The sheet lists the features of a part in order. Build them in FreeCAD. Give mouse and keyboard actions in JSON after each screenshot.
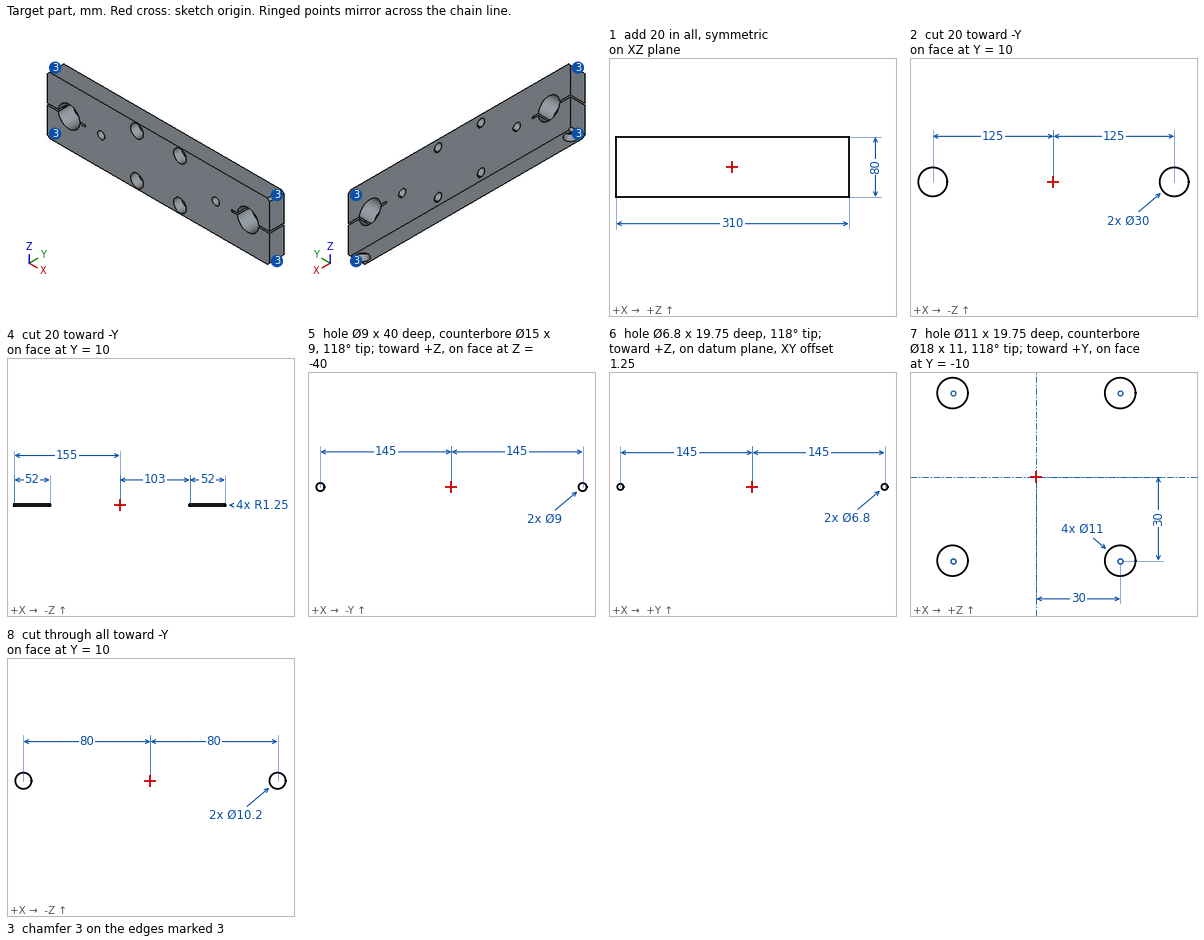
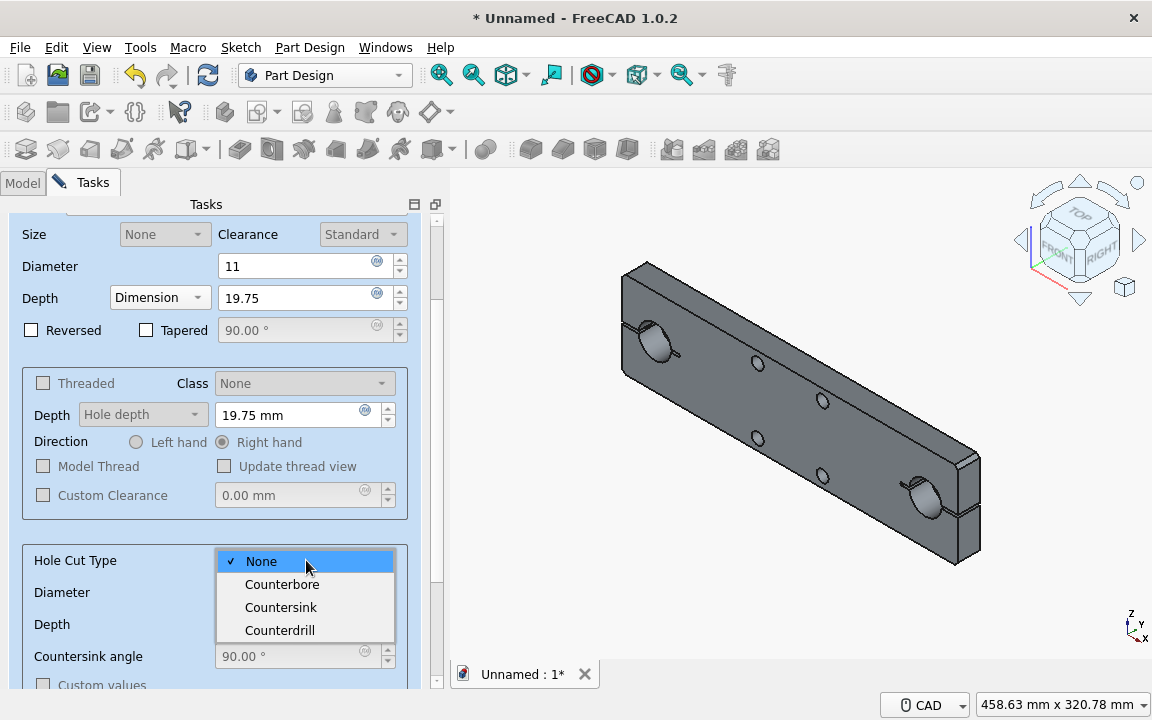
{"action": "left_click", "coordinate": [304, 584]}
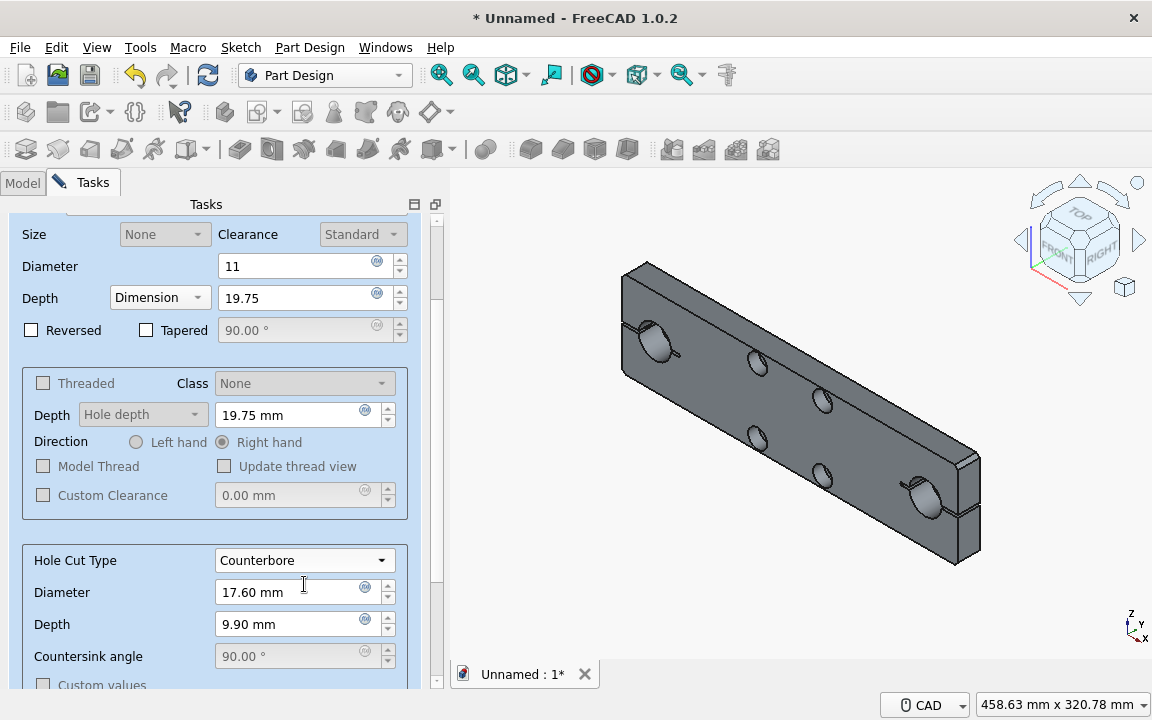
{"action": "triple_click", "coordinate": [298, 592]}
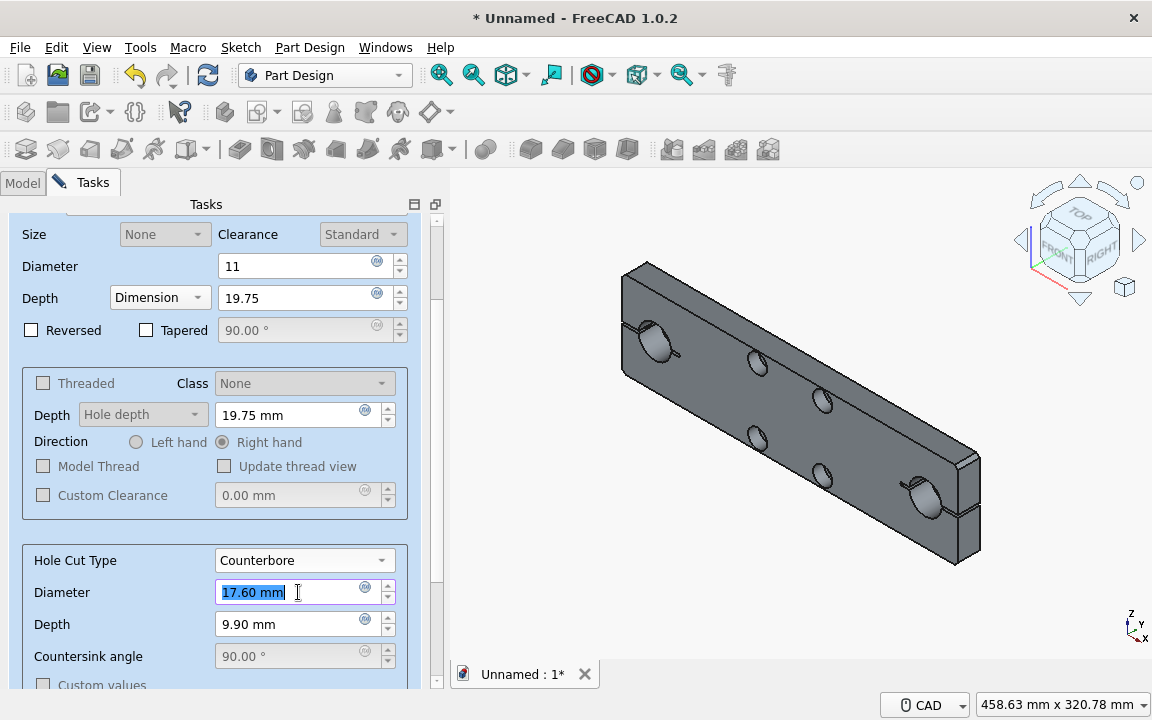
{"action": "type", "text": "18"}
{"action": "key", "text": "Tab"}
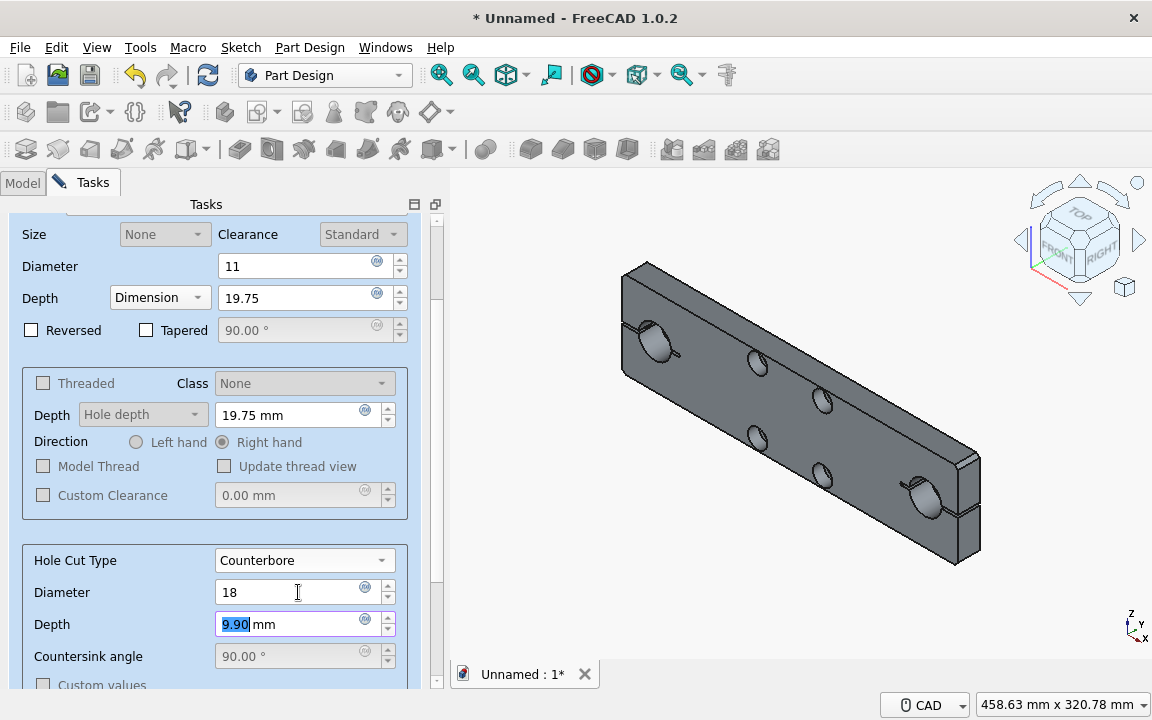
{"action": "type", "text": "11"}
{"action": "key", "text": "Tab"}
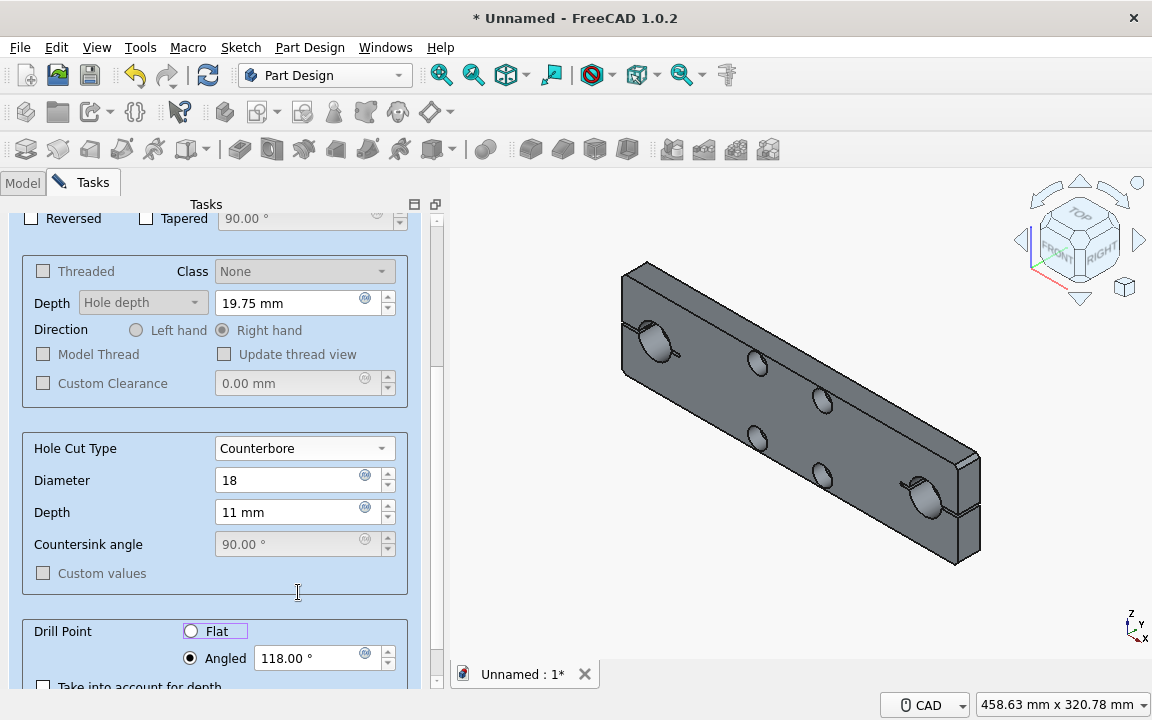
{"action": "scroll", "coordinate": [437, 451], "scroll_direction": "up", "scroll_amount": 5}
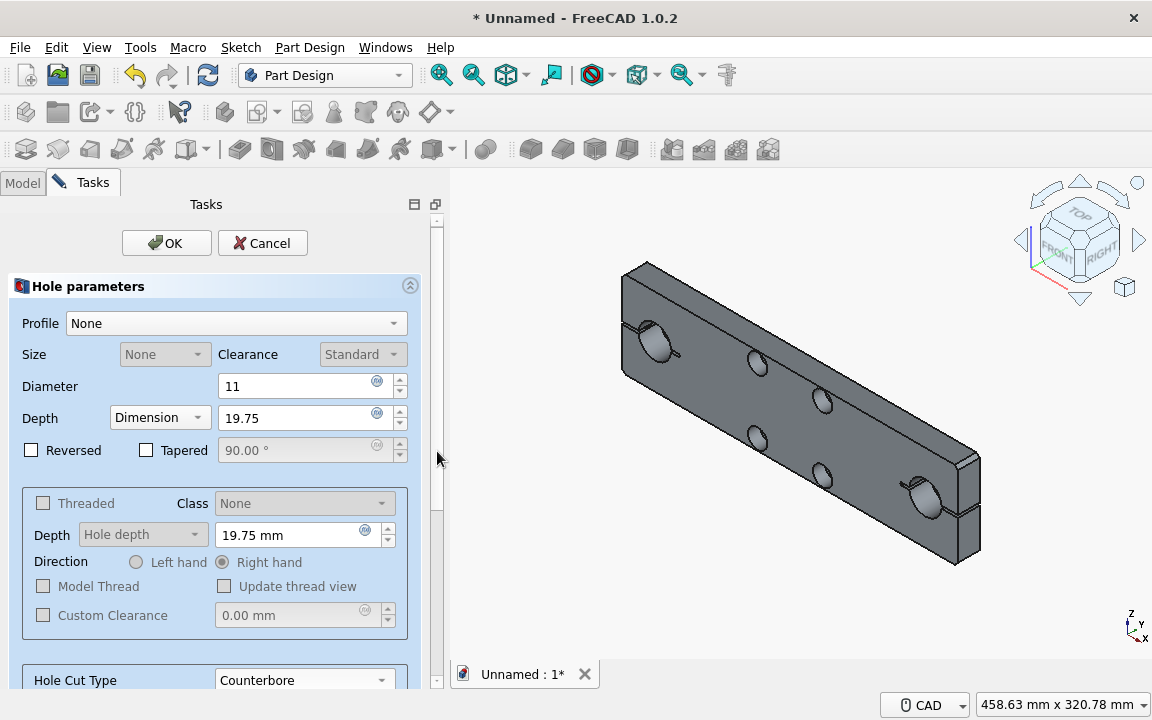
{"action": "left_click", "coordinate": [167, 243]}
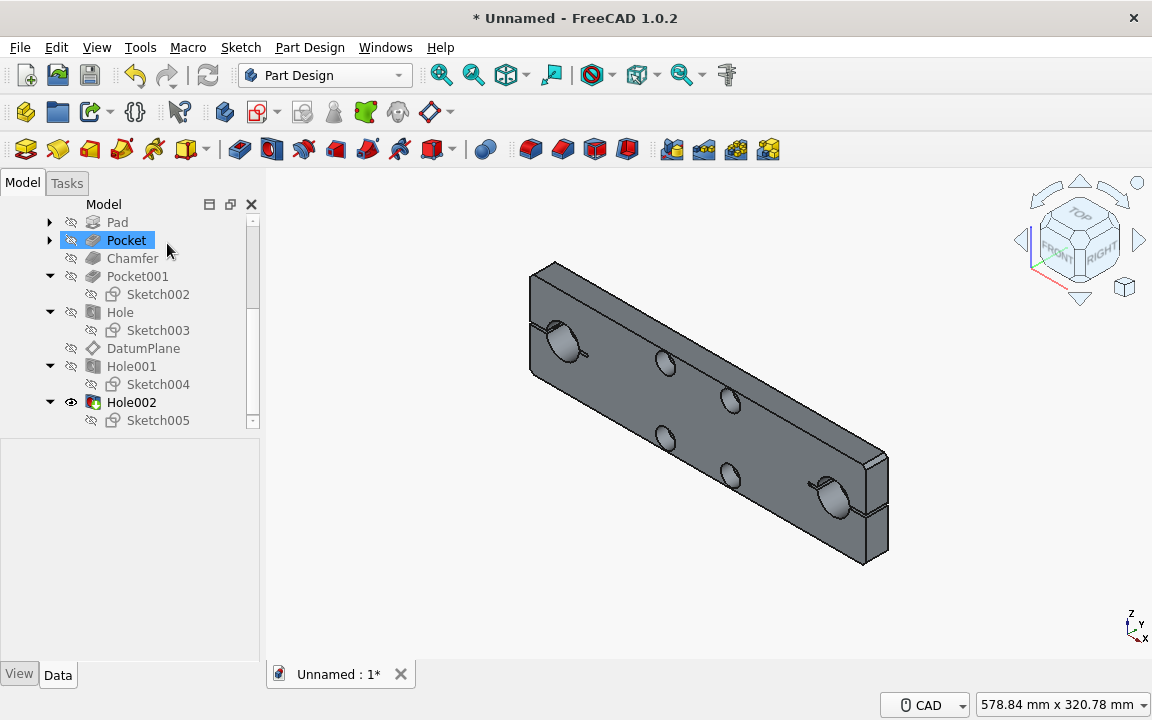
{"action": "key", "text": "4"}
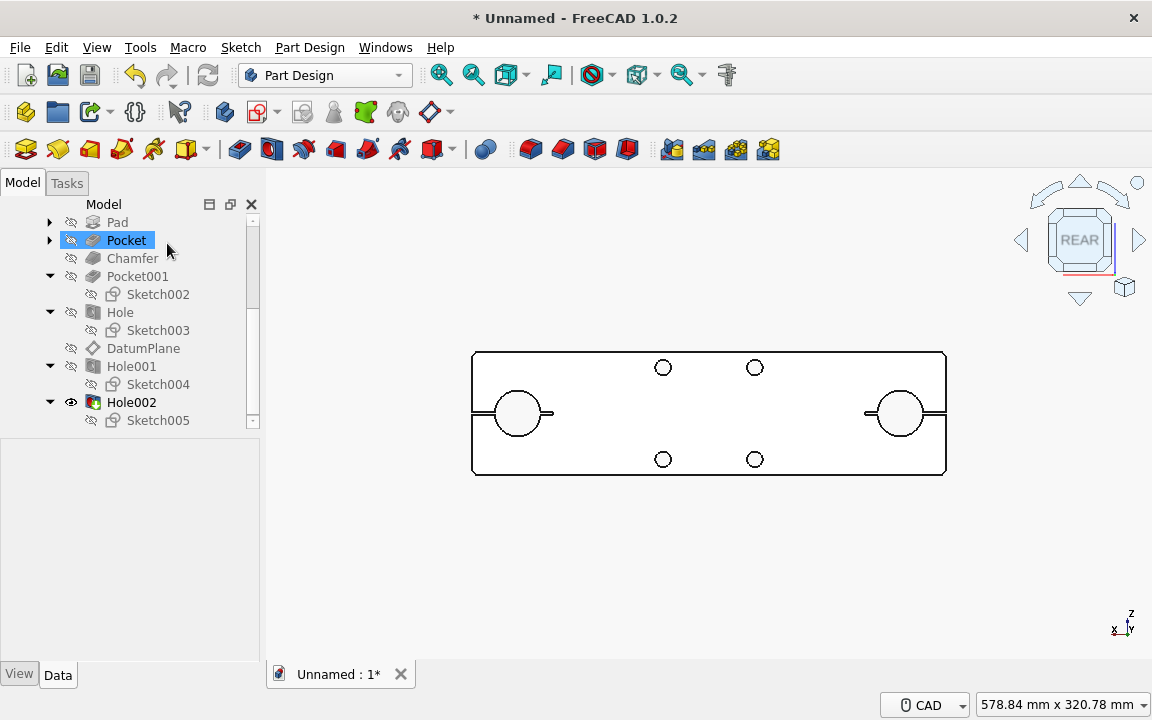
{"action": "left_click", "coordinate": [709, 412]}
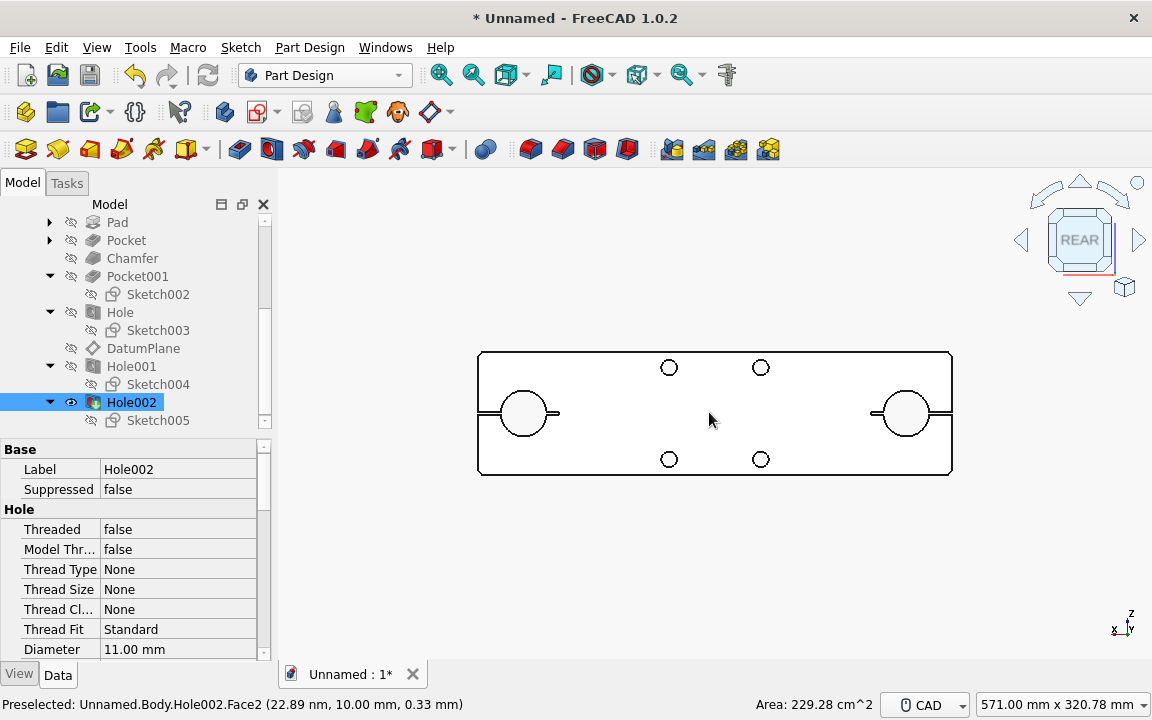
{"action": "left_click", "coordinate": [258, 112]}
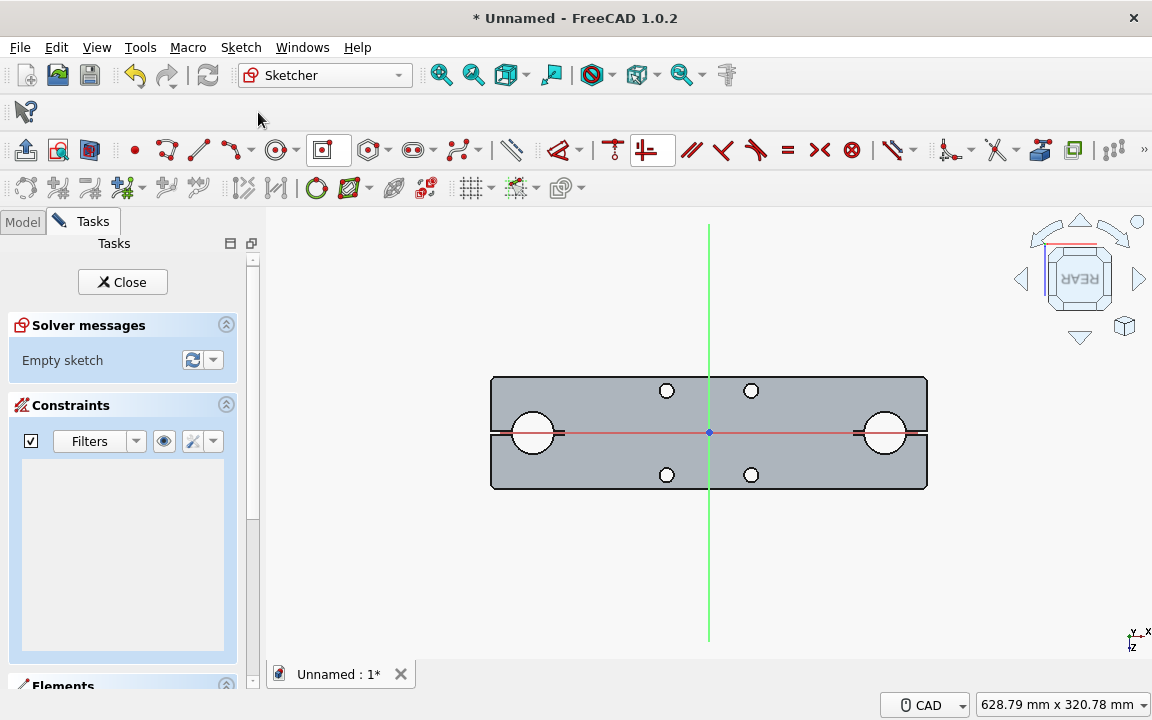
{"action": "scroll", "coordinate": [765, 433], "scroll_direction": "up", "scroll_amount": 4}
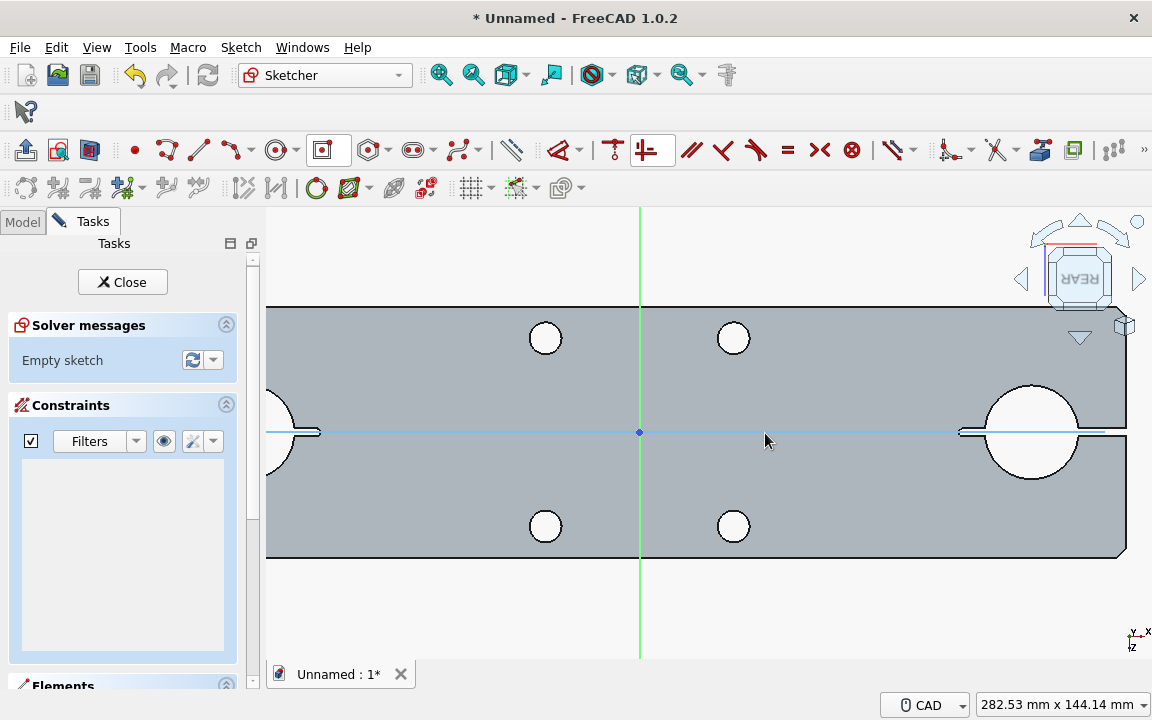
{"action": "left_click", "coordinate": [276, 150]}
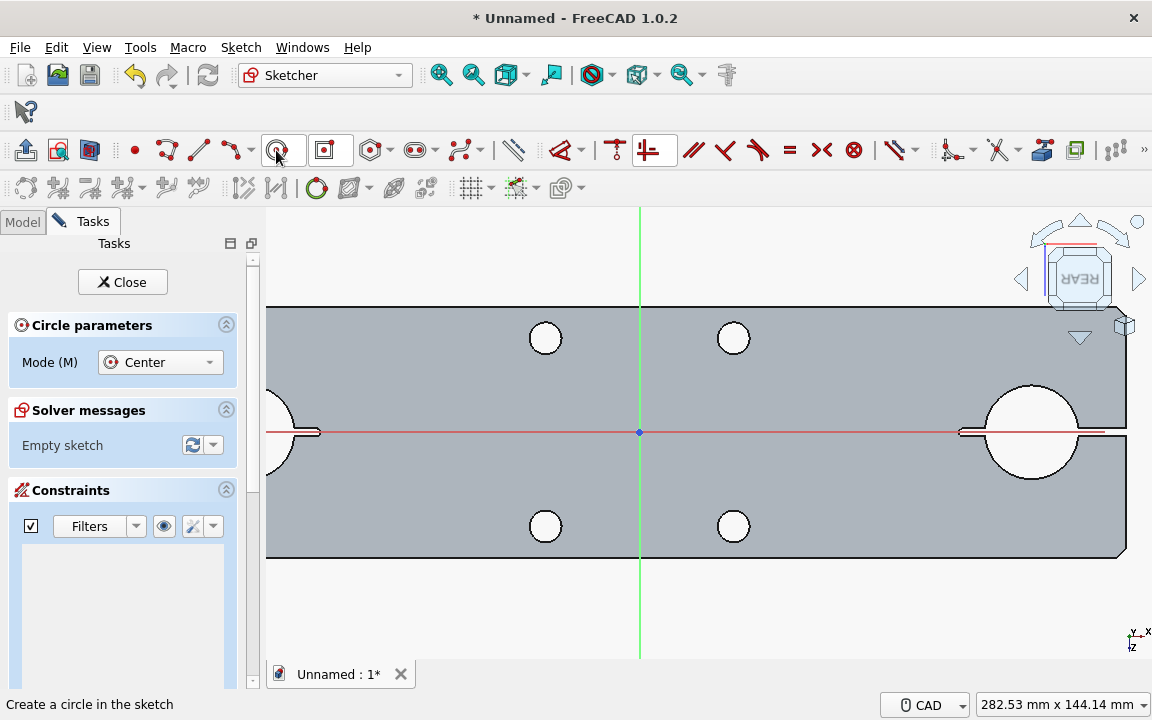
{"action": "scroll", "coordinate": [891, 432], "scroll_direction": "up", "scroll_amount": 2}